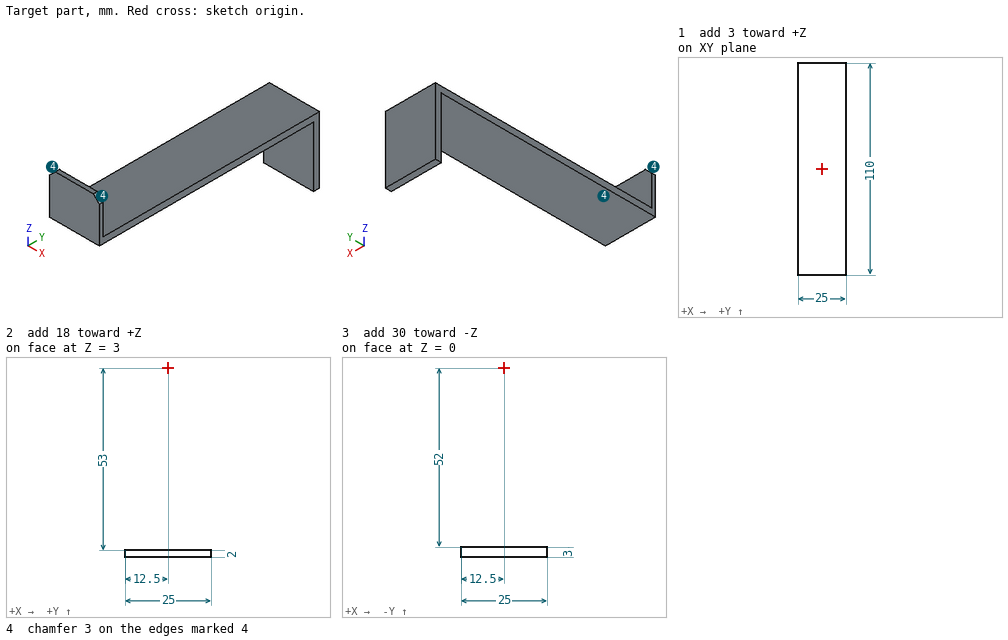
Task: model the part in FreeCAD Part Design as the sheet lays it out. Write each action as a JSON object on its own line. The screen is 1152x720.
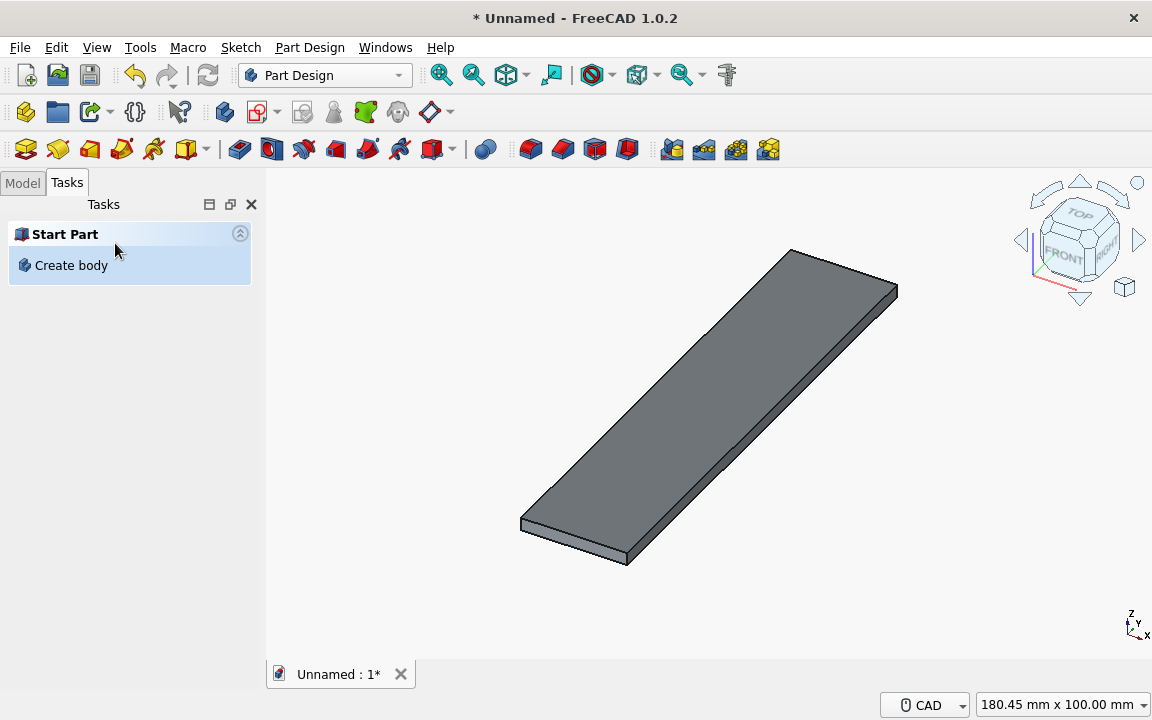
{"action": "left_click", "coordinate": [786, 324]}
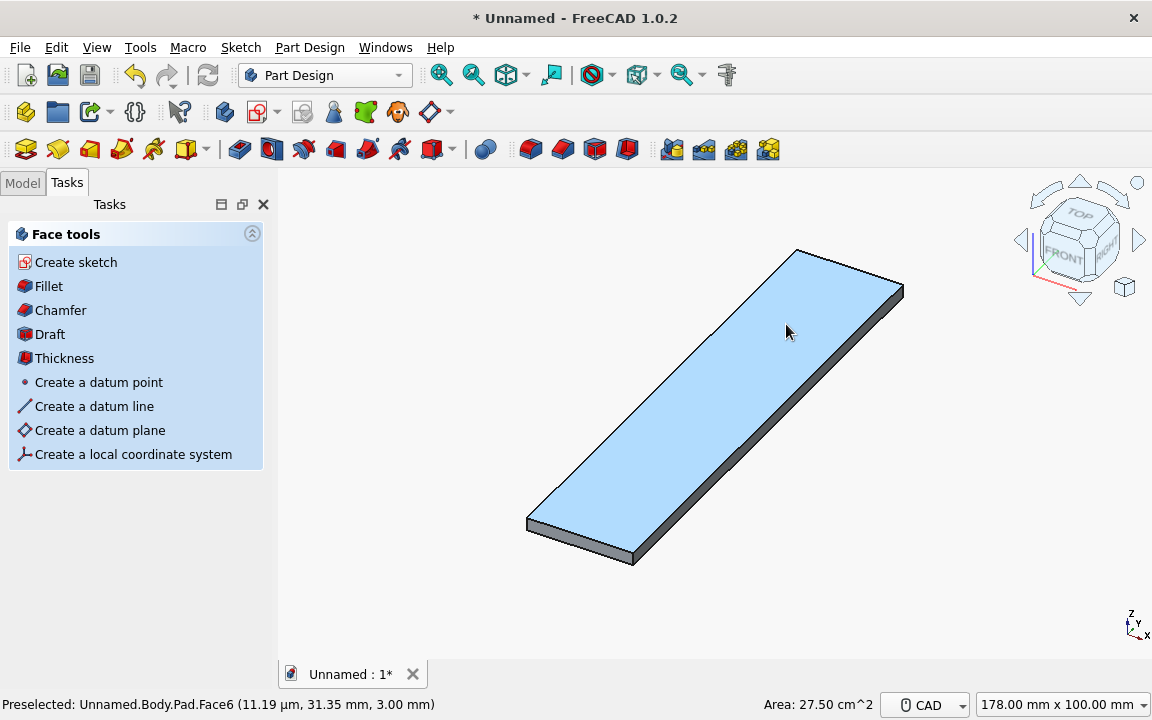
{"action": "left_click", "coordinate": [258, 112]}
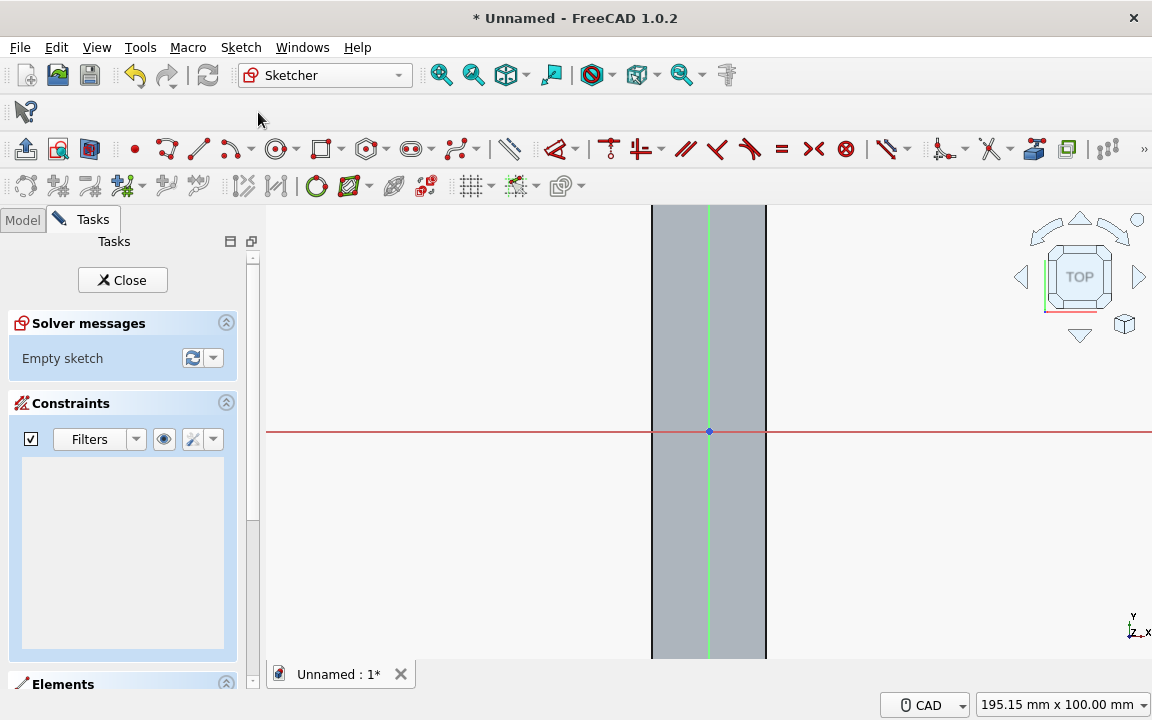
{"action": "scroll", "coordinate": [331, 233], "scroll_direction": "down", "scroll_amount": 1}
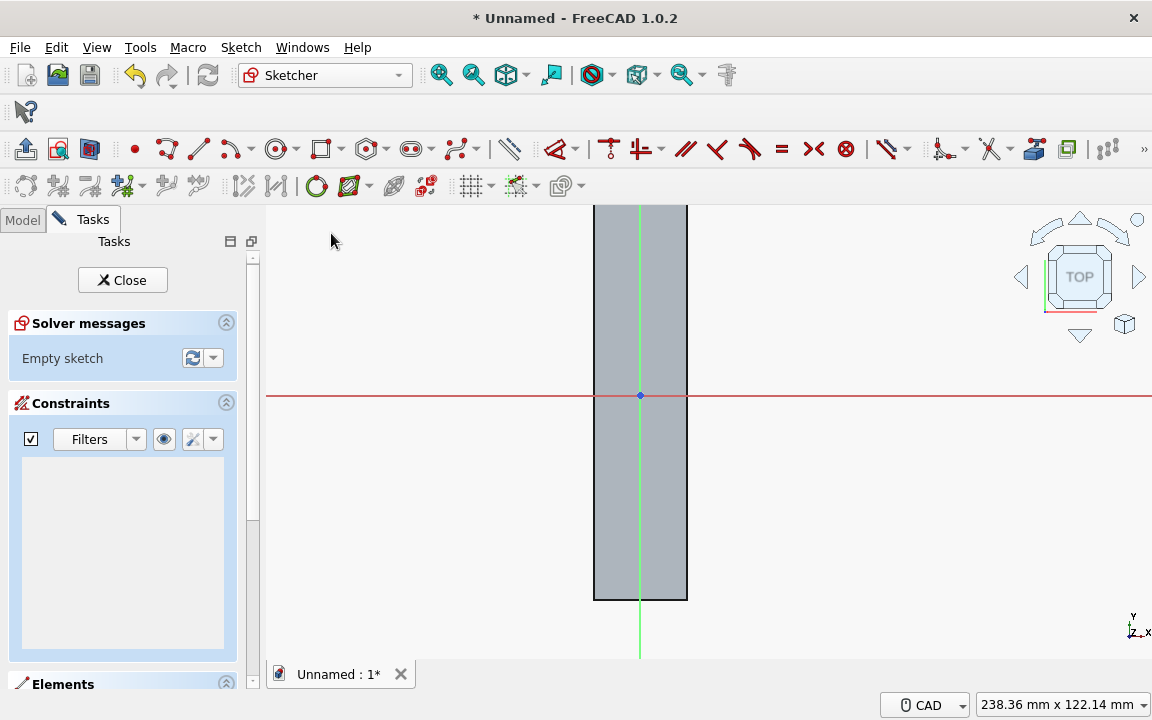
{"action": "scroll", "coordinate": [640, 631], "scroll_direction": "up", "scroll_amount": 2}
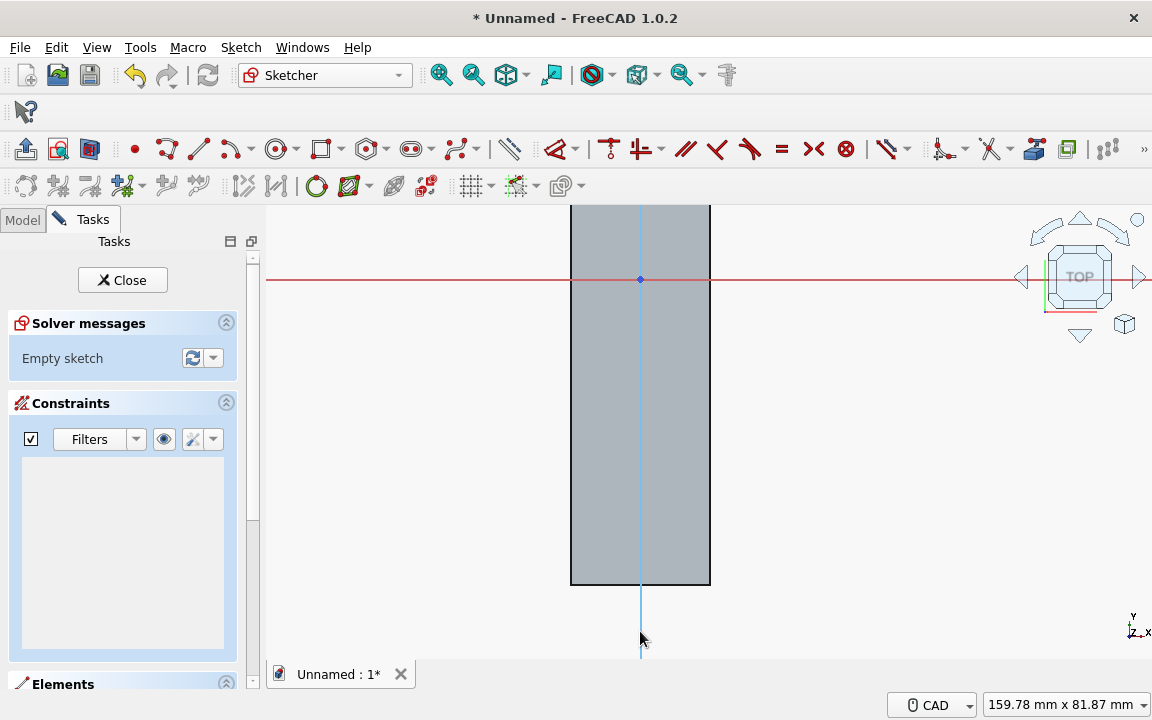
{"action": "key", "text": "g r"}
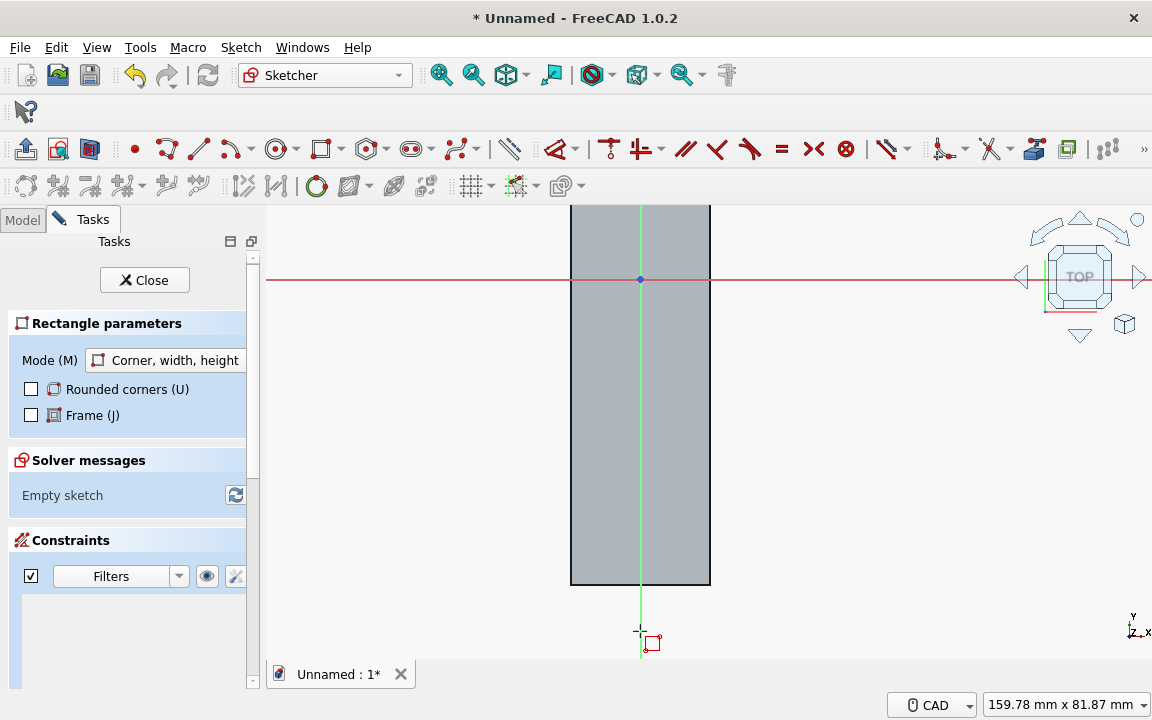
{"action": "scroll", "coordinate": [571, 574], "scroll_direction": "up", "scroll_amount": 2}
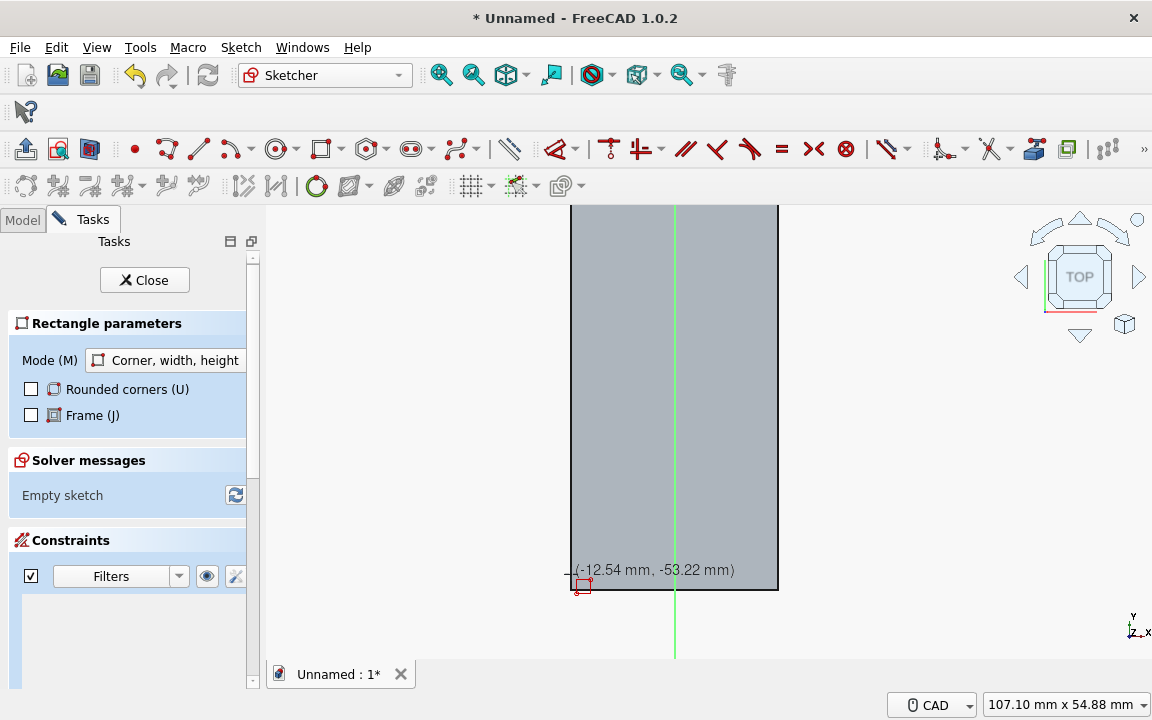
{"action": "left_click", "coordinate": [571, 573]}
{"action": "mouse_move", "coordinate": [778, 590]}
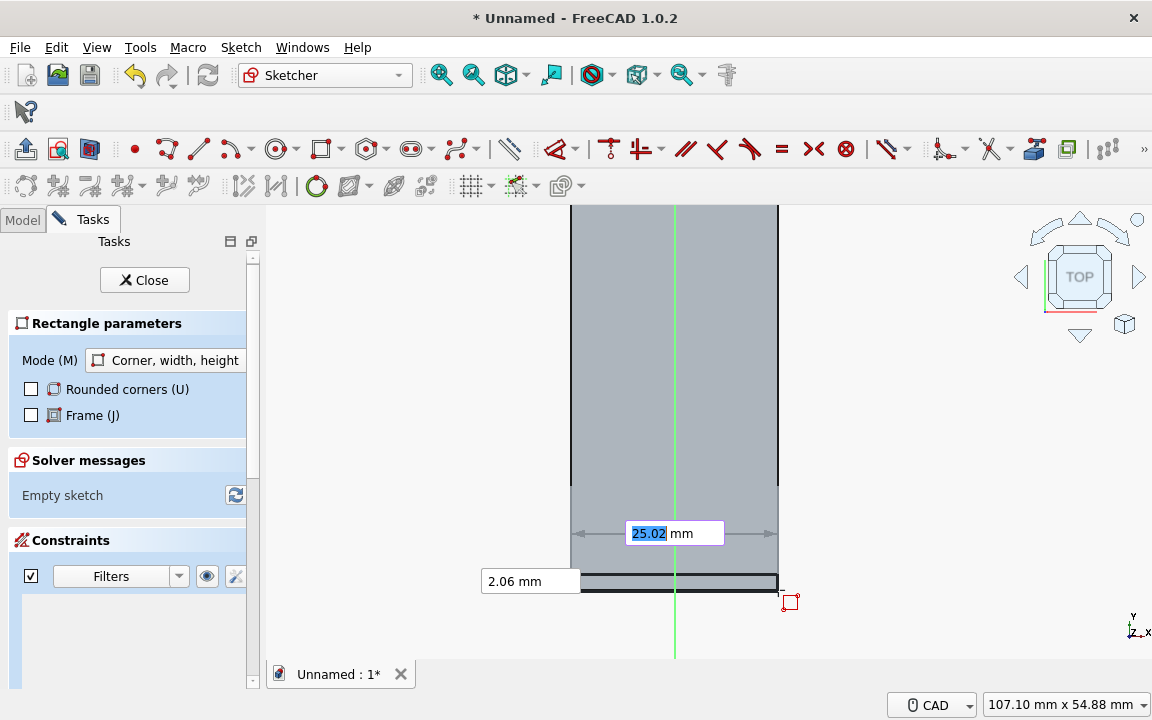
{"action": "type", "text": "25"}
{"action": "key", "text": "Tab"}
{"action": "type", "text": "2"}
{"action": "key", "text": "Return"}
{"action": "key", "text": "Escape"}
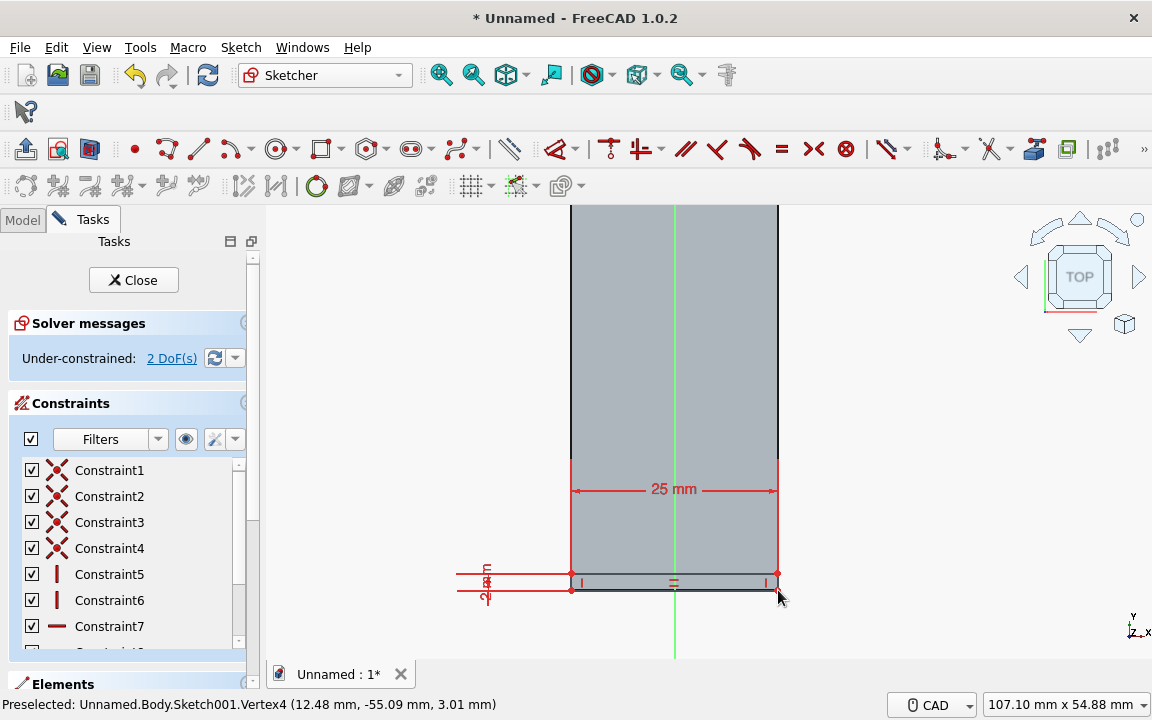
{"action": "key", "text": "d"}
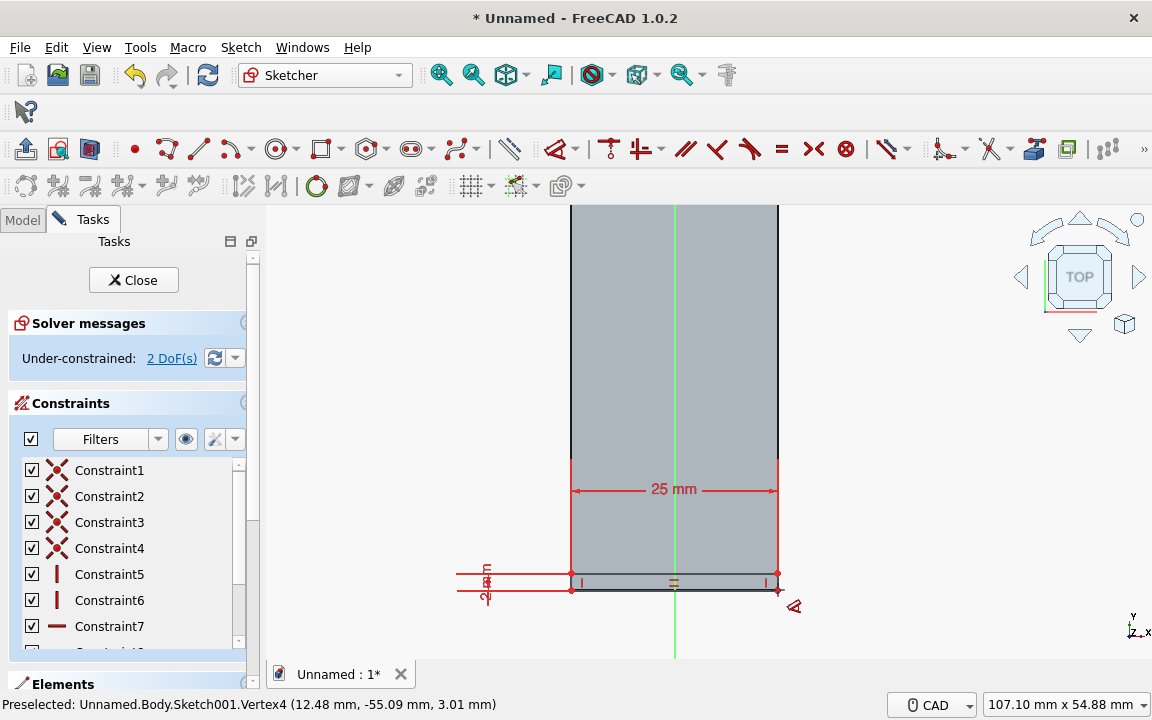
{"action": "left_click", "coordinate": [571, 574]}
{"action": "left_click", "coordinate": [537, 403]}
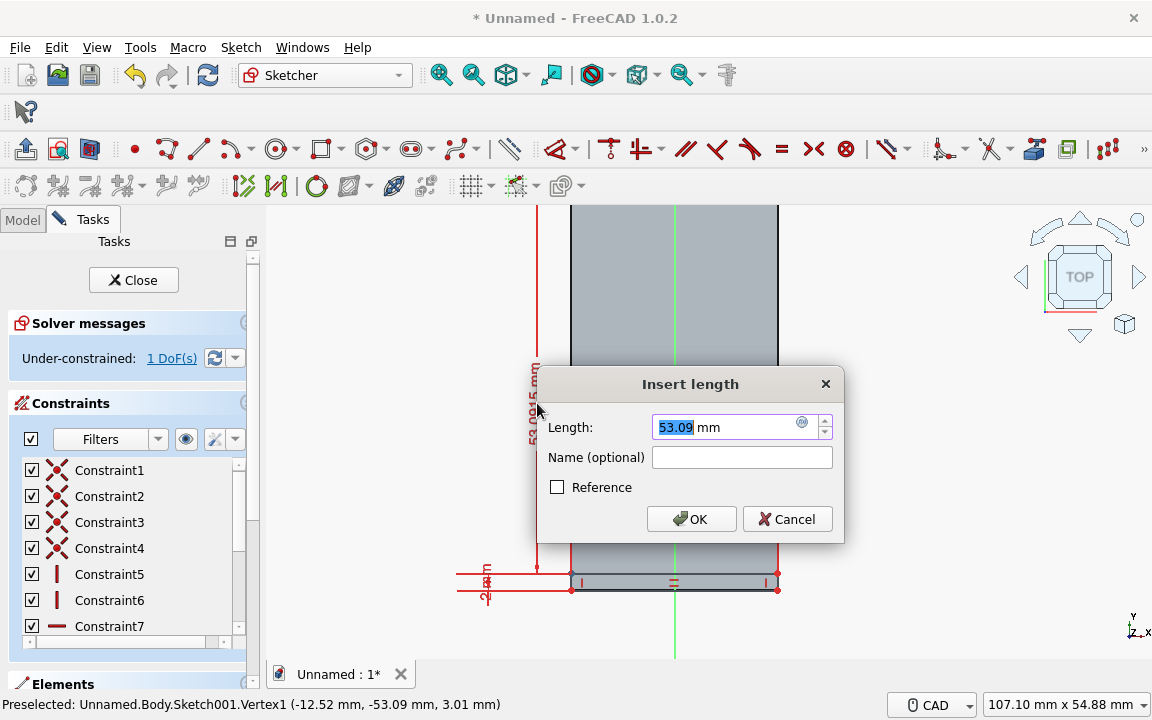
{"action": "type", "text": "53"}
{"action": "key", "text": "Return"}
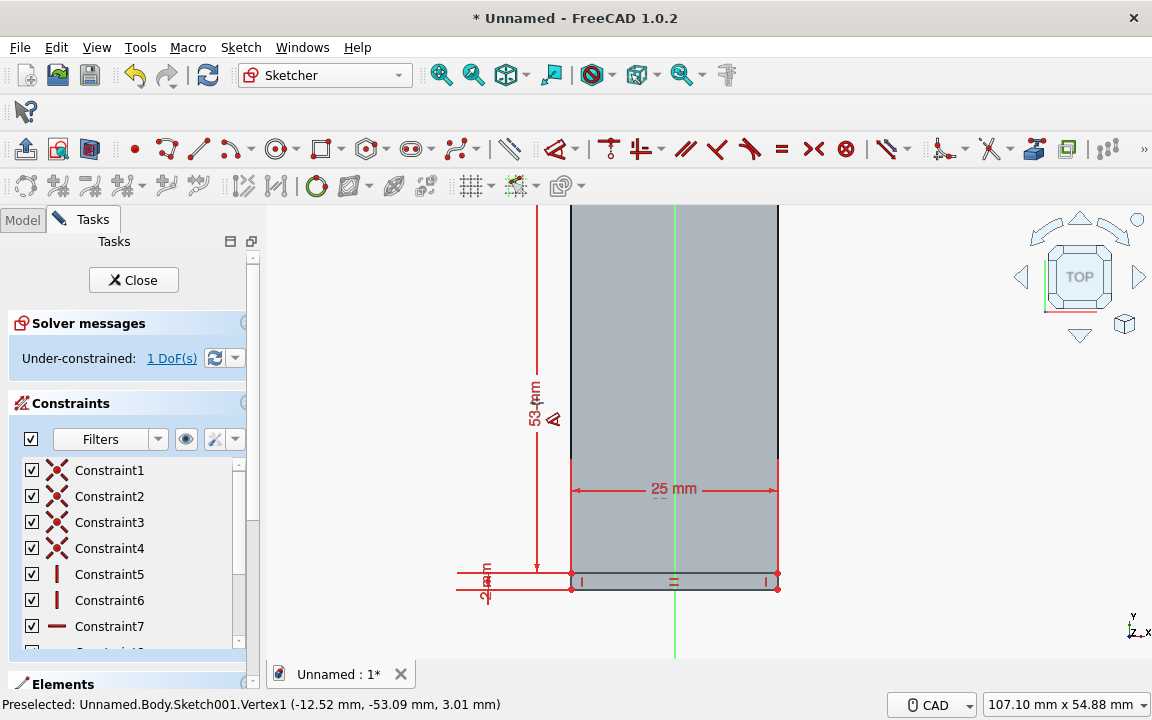
{"action": "left_click", "coordinate": [571, 573]}
{"action": "left_click", "coordinate": [623, 607]}